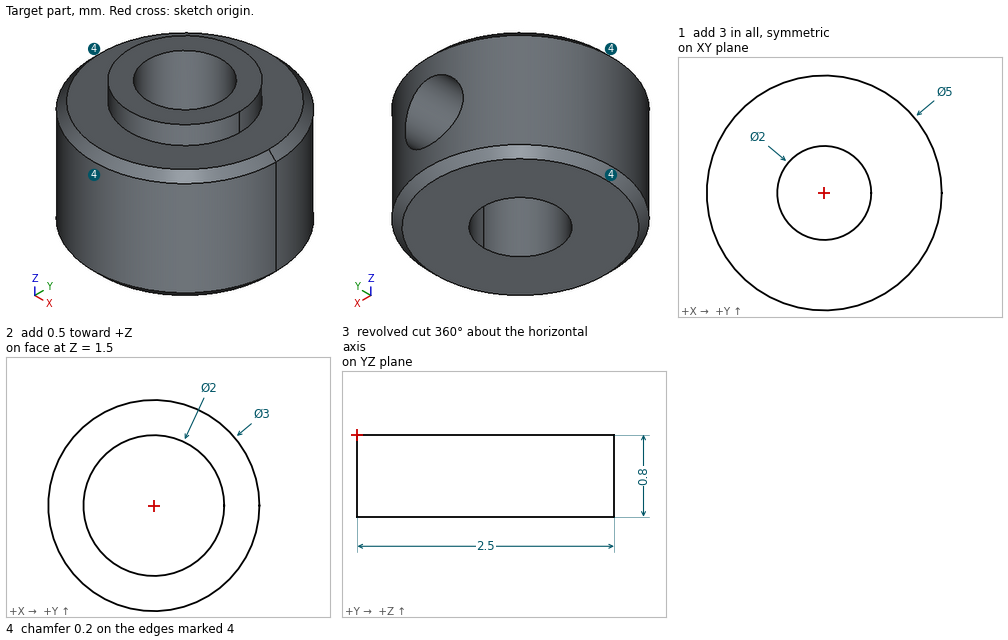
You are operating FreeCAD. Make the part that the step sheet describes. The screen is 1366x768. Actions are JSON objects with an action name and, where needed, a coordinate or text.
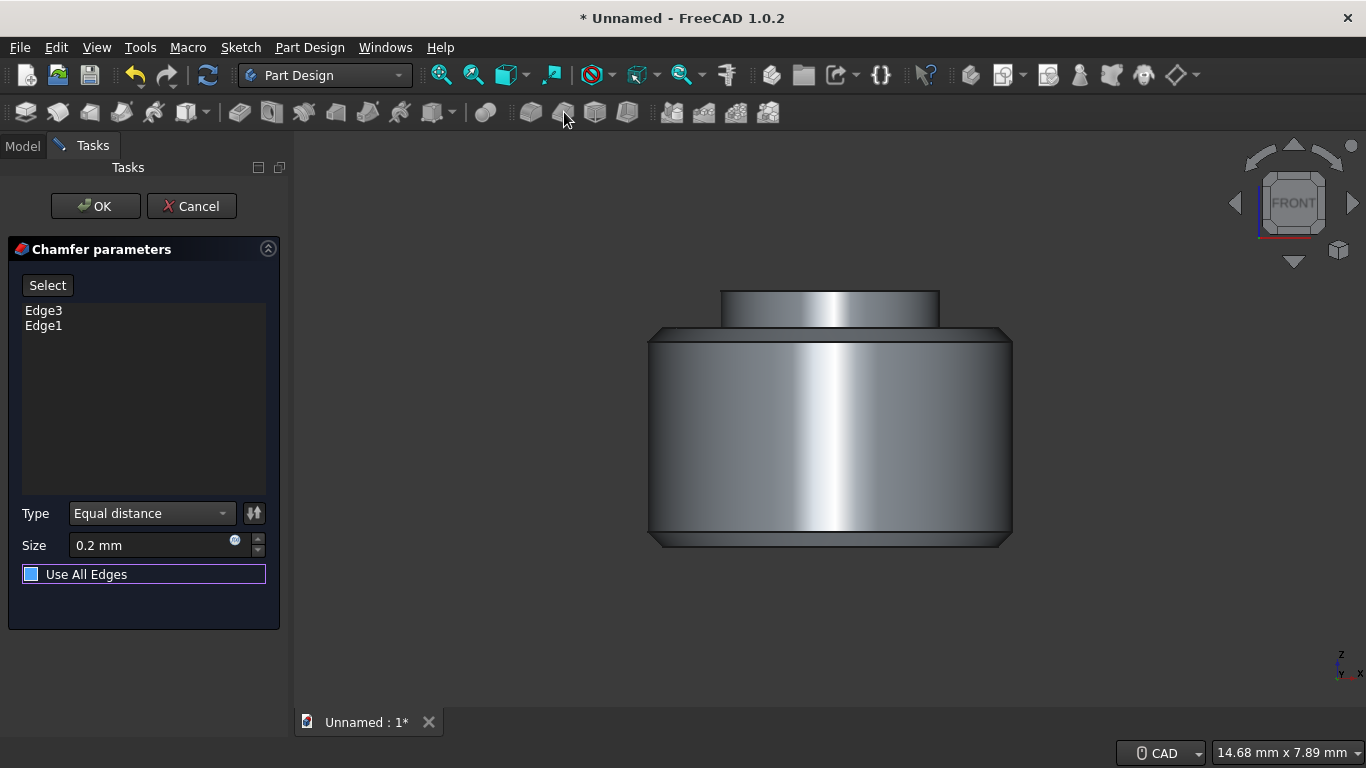
{"action": "left_click", "coordinate": [96, 206]}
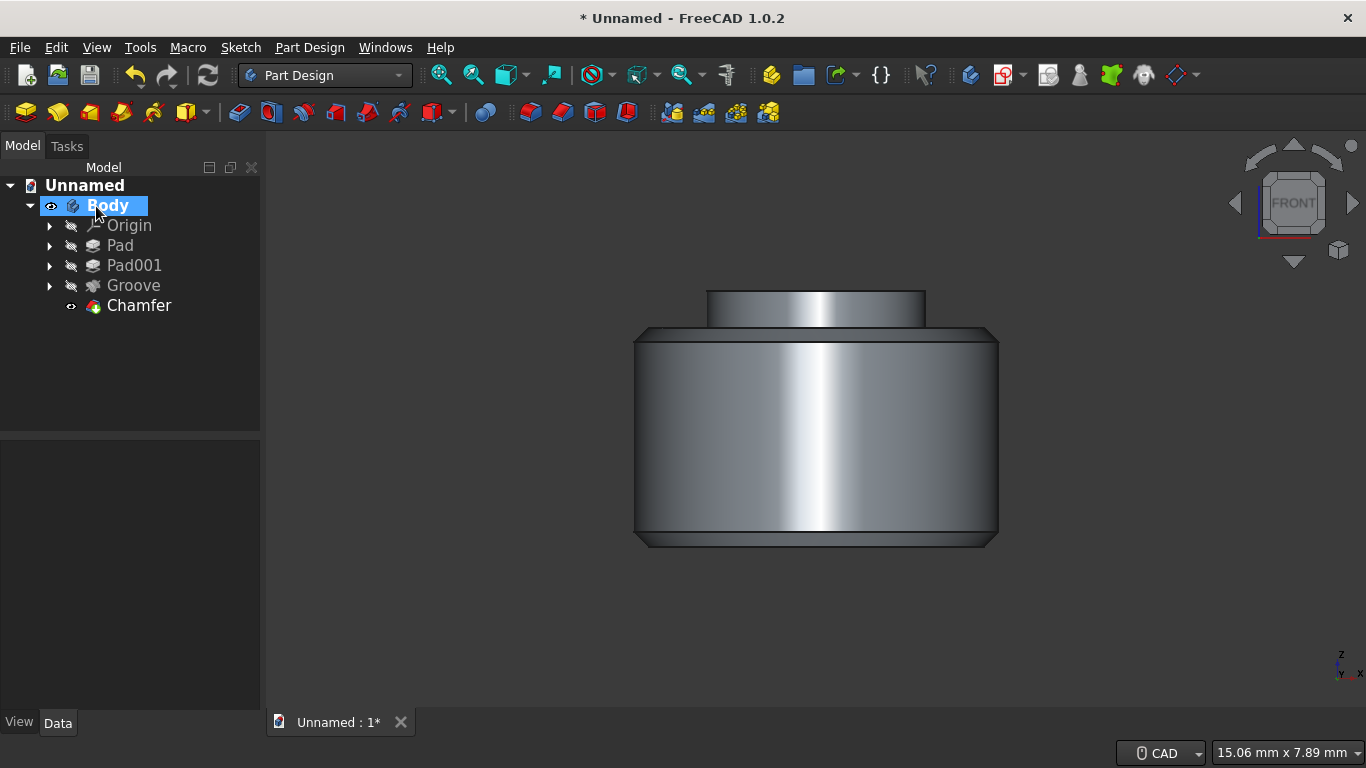
{"action": "key", "text": "0"}